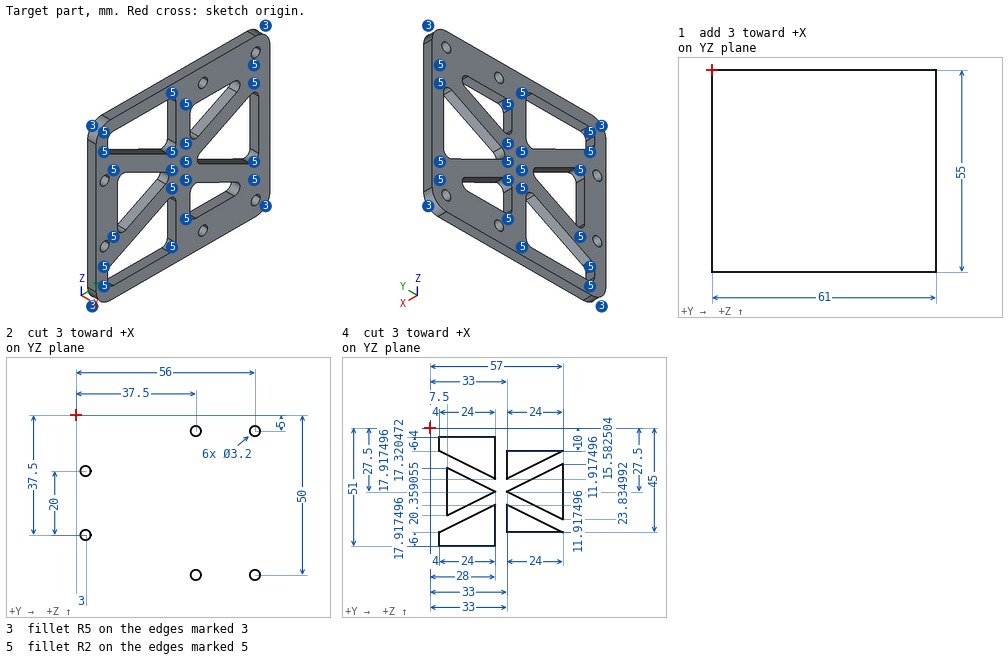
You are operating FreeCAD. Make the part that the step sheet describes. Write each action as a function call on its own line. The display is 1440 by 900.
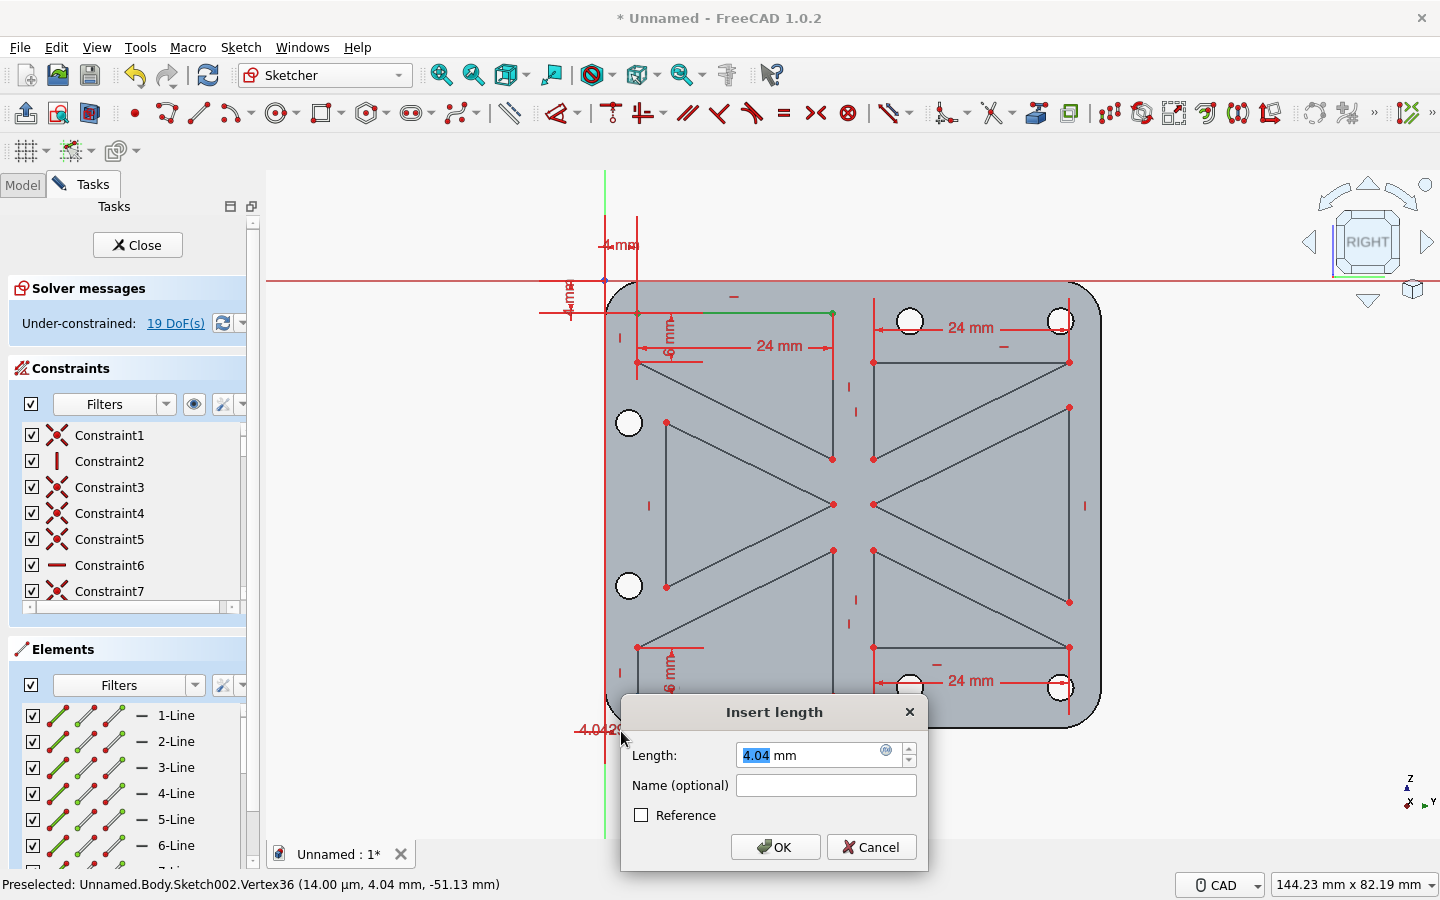
text(4)
key(Return)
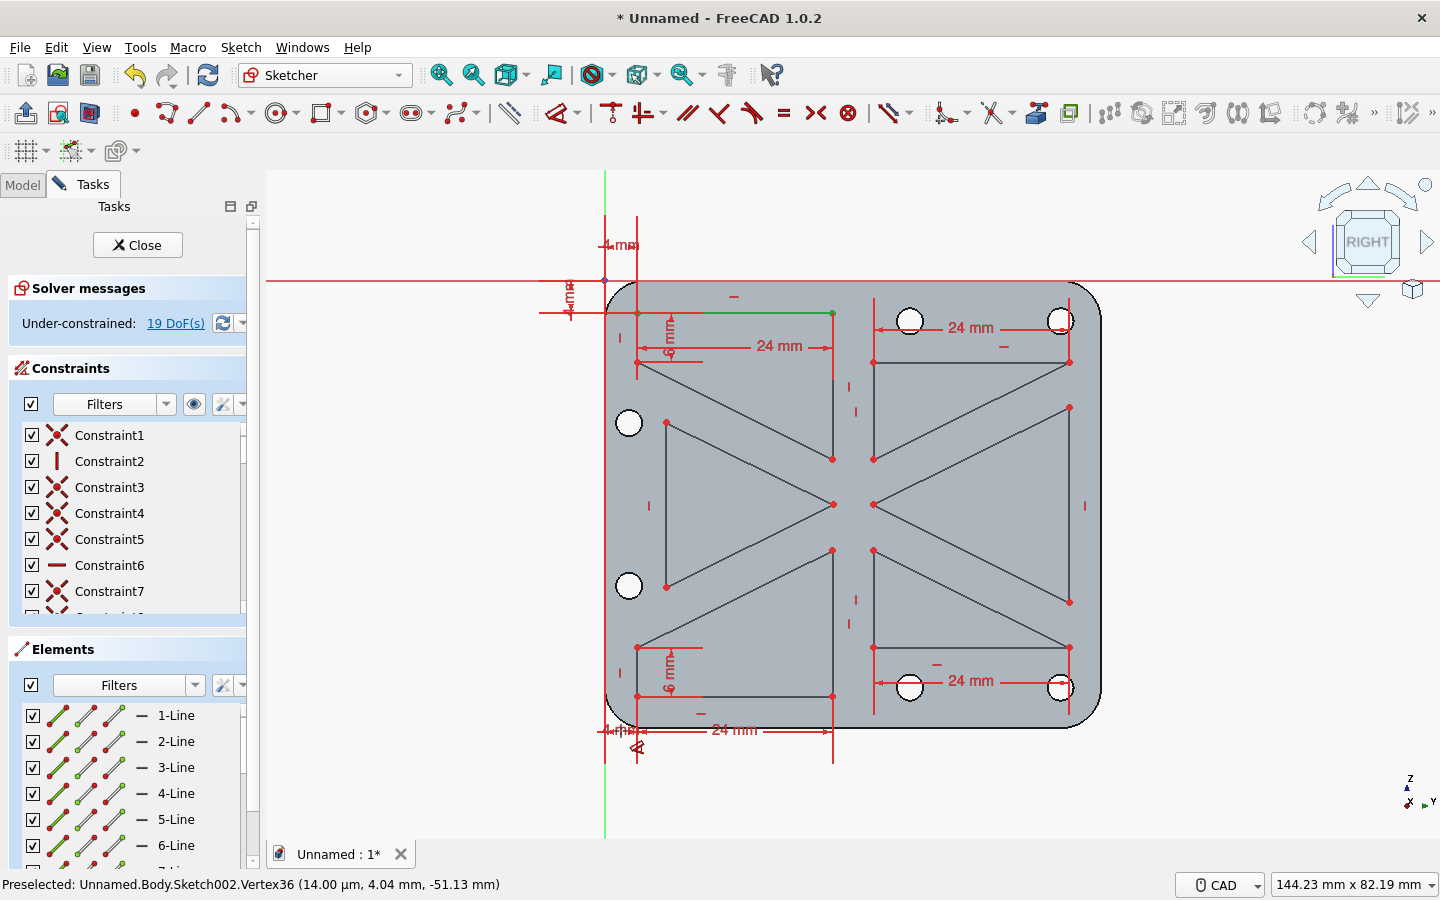
click(873, 505)
click(739, 247)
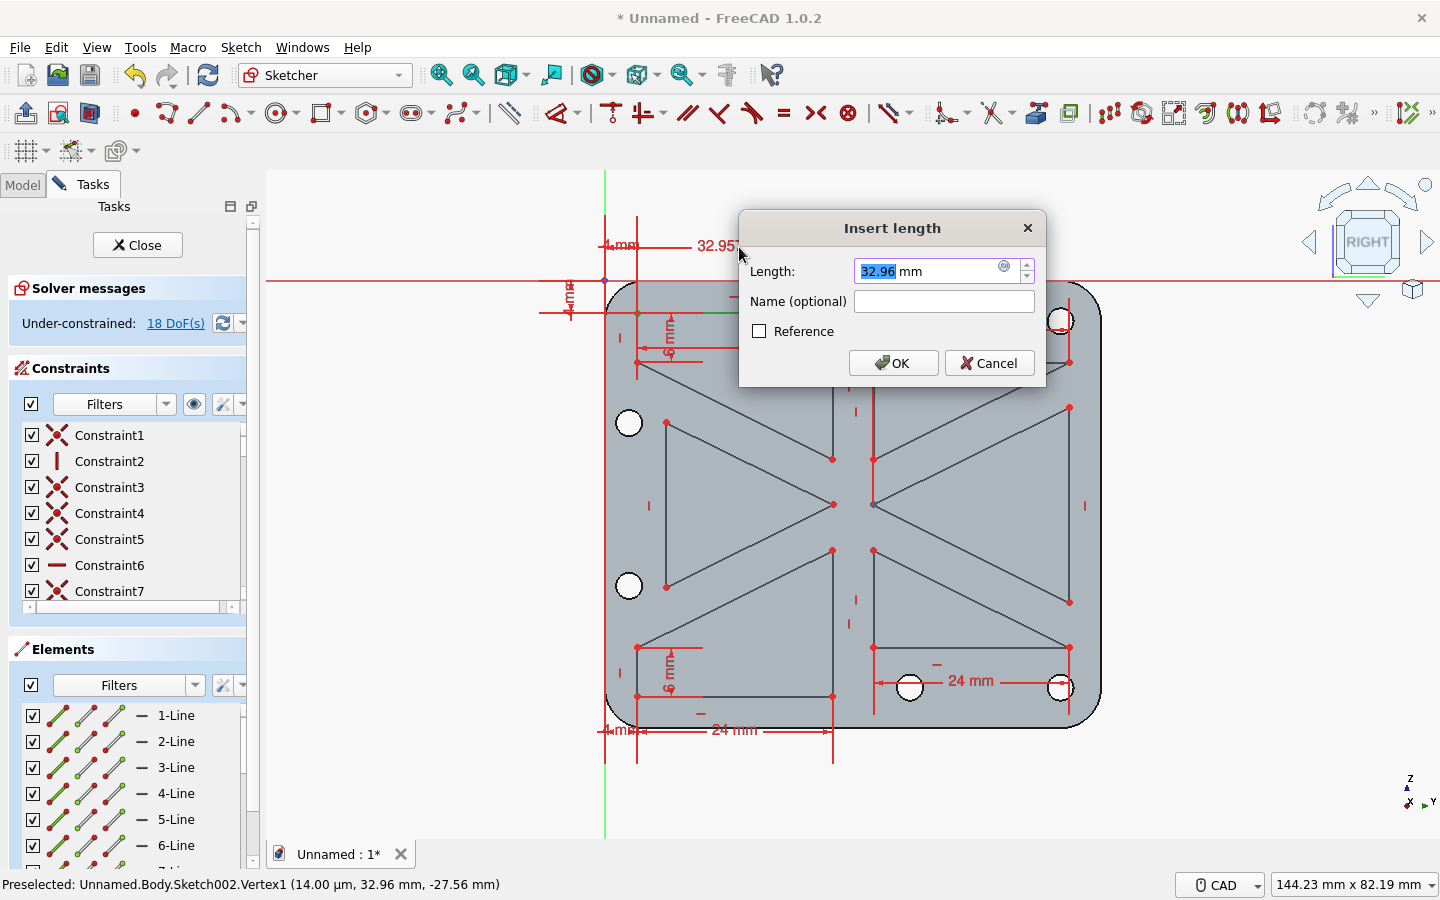
text(33)
key(Return)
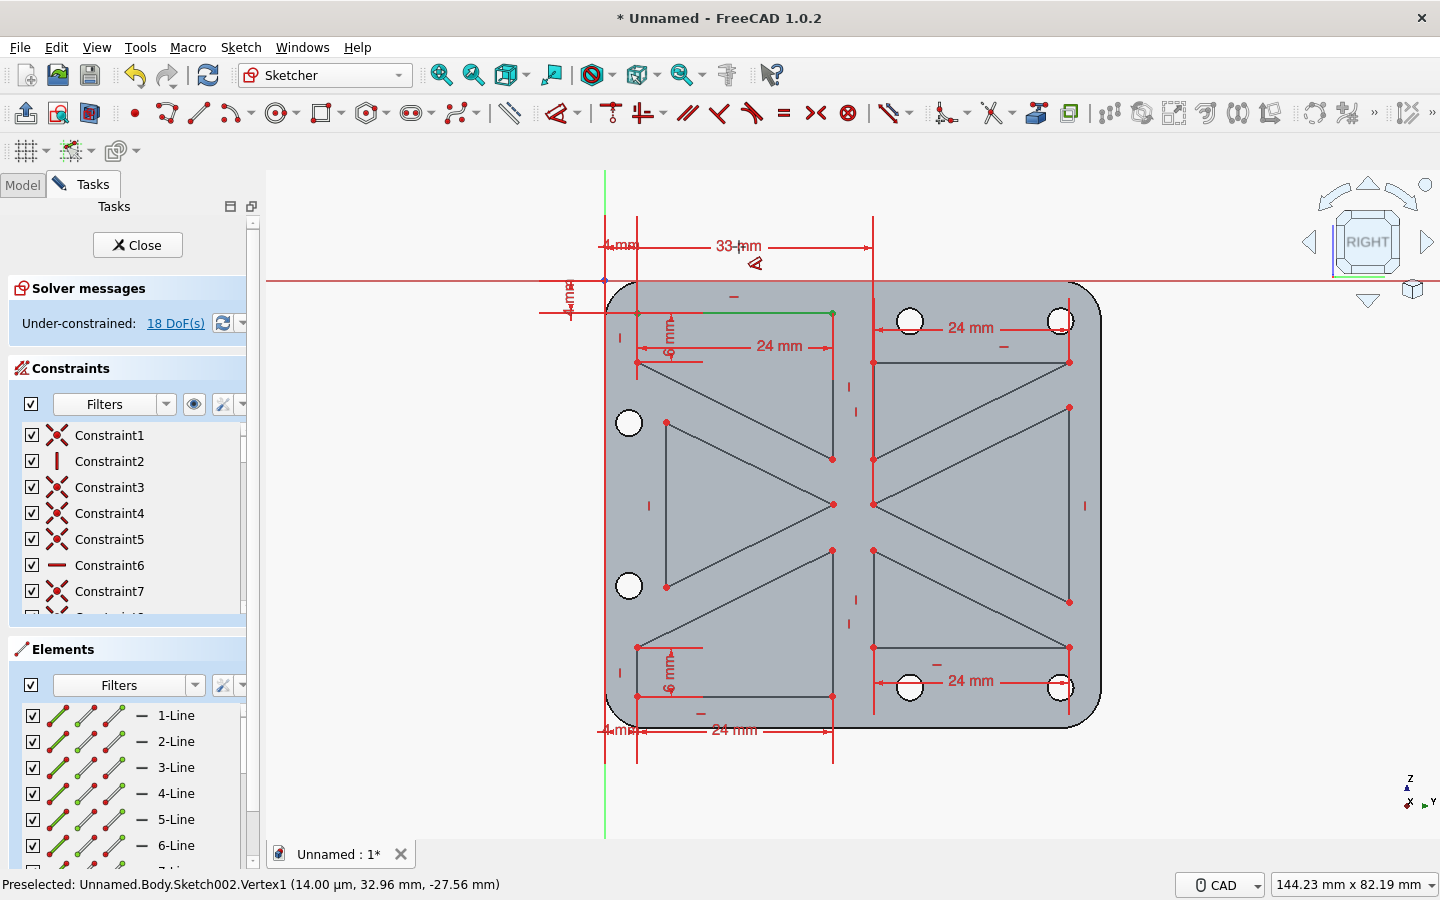
click(1069, 408)
click(837, 247)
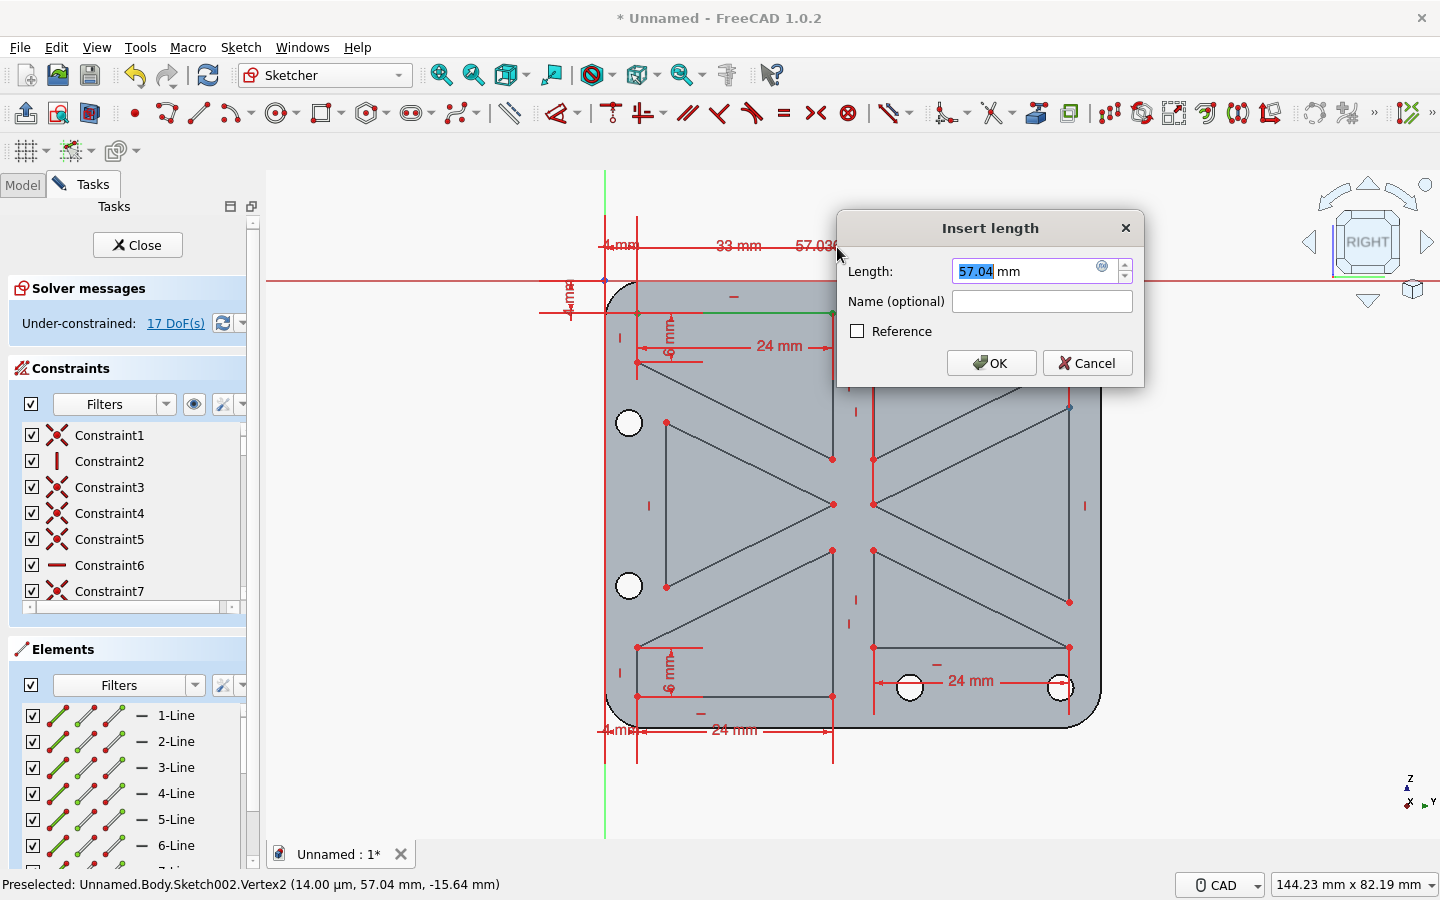
text(57)
key(Return)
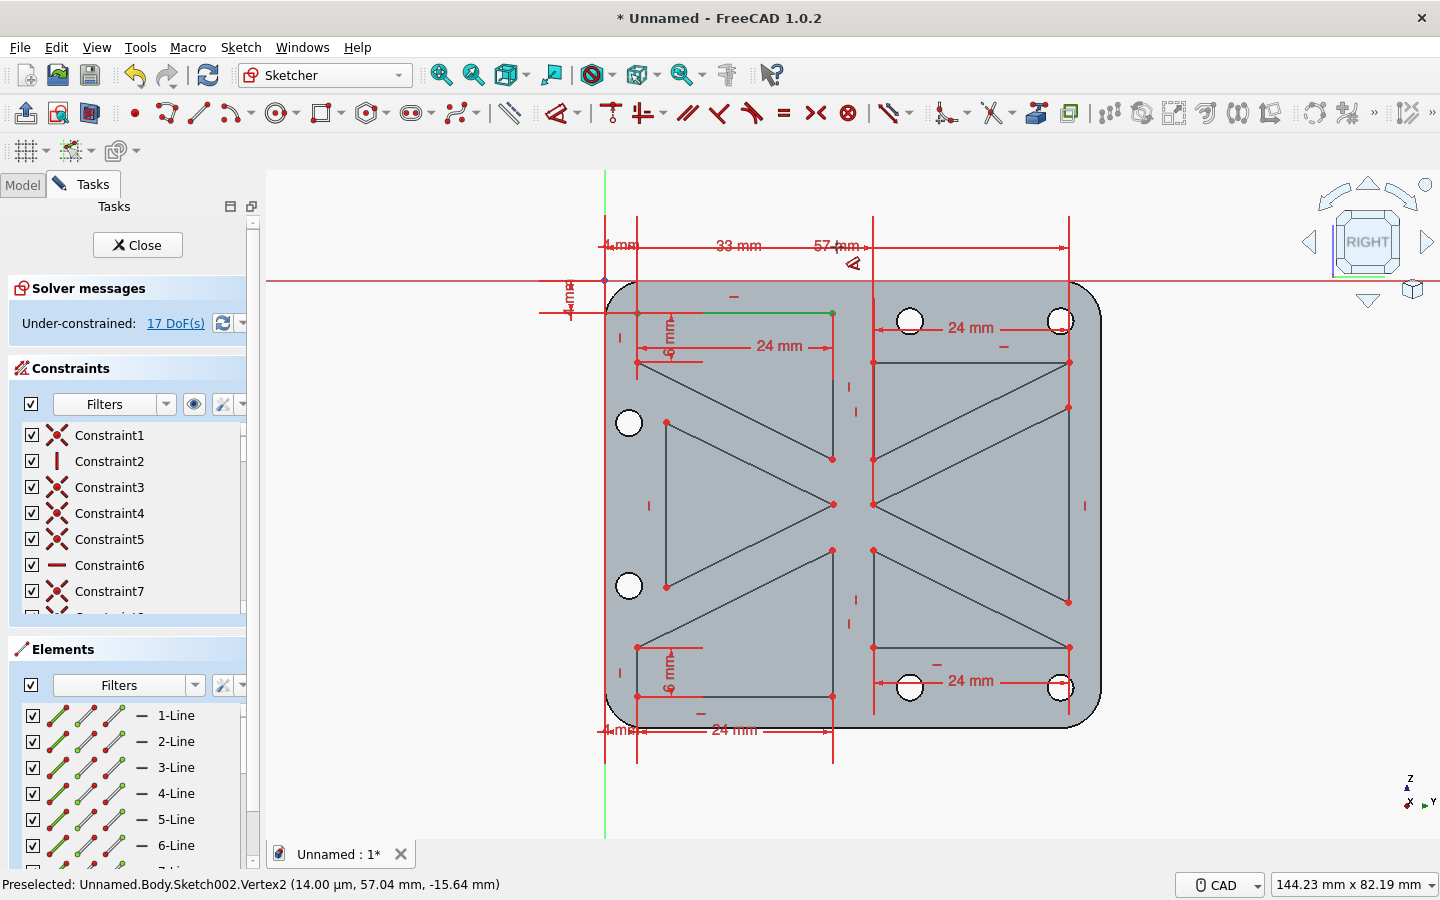
click(874, 551)
click(801, 585)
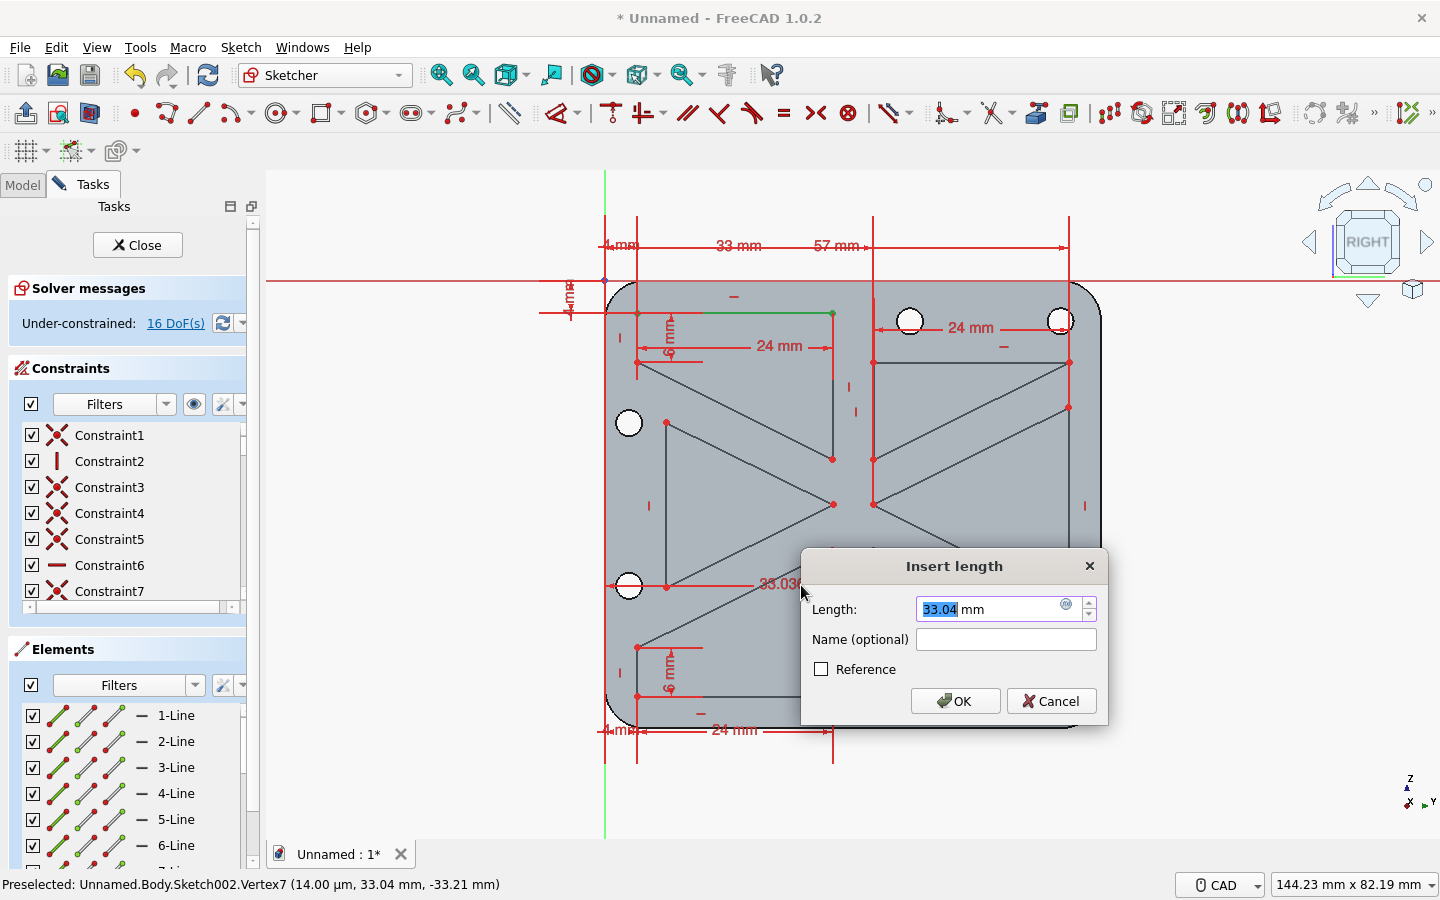
text(33)
key(Return)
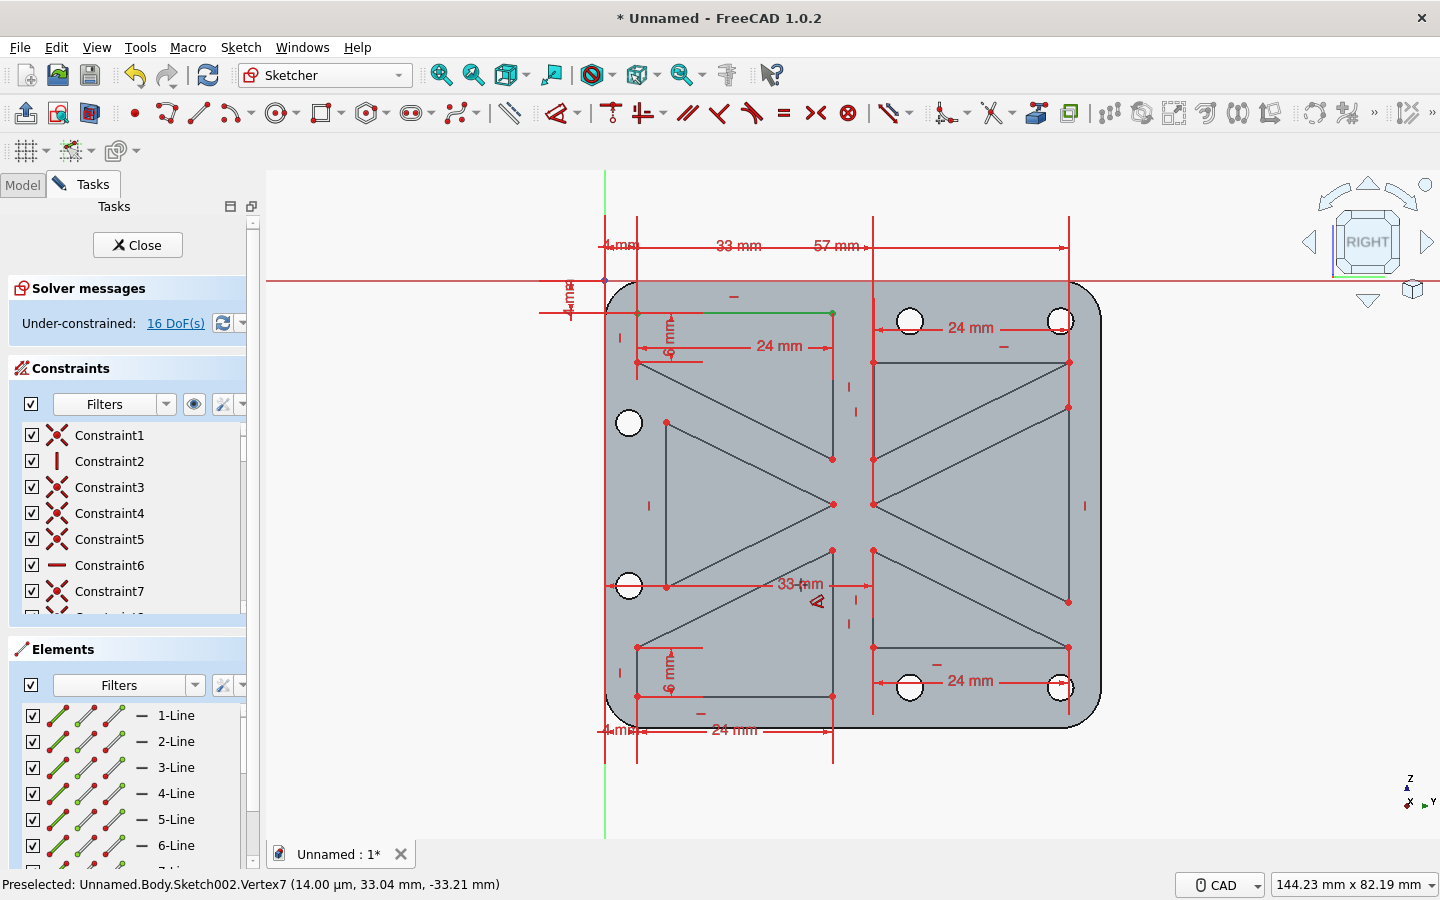
click(1069, 648)
click(1103, 464)